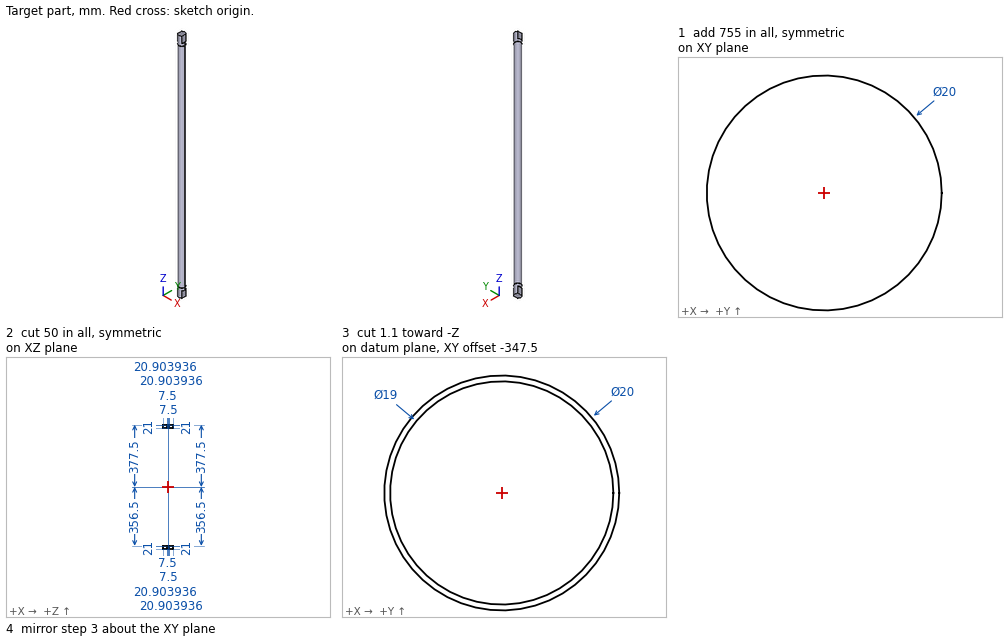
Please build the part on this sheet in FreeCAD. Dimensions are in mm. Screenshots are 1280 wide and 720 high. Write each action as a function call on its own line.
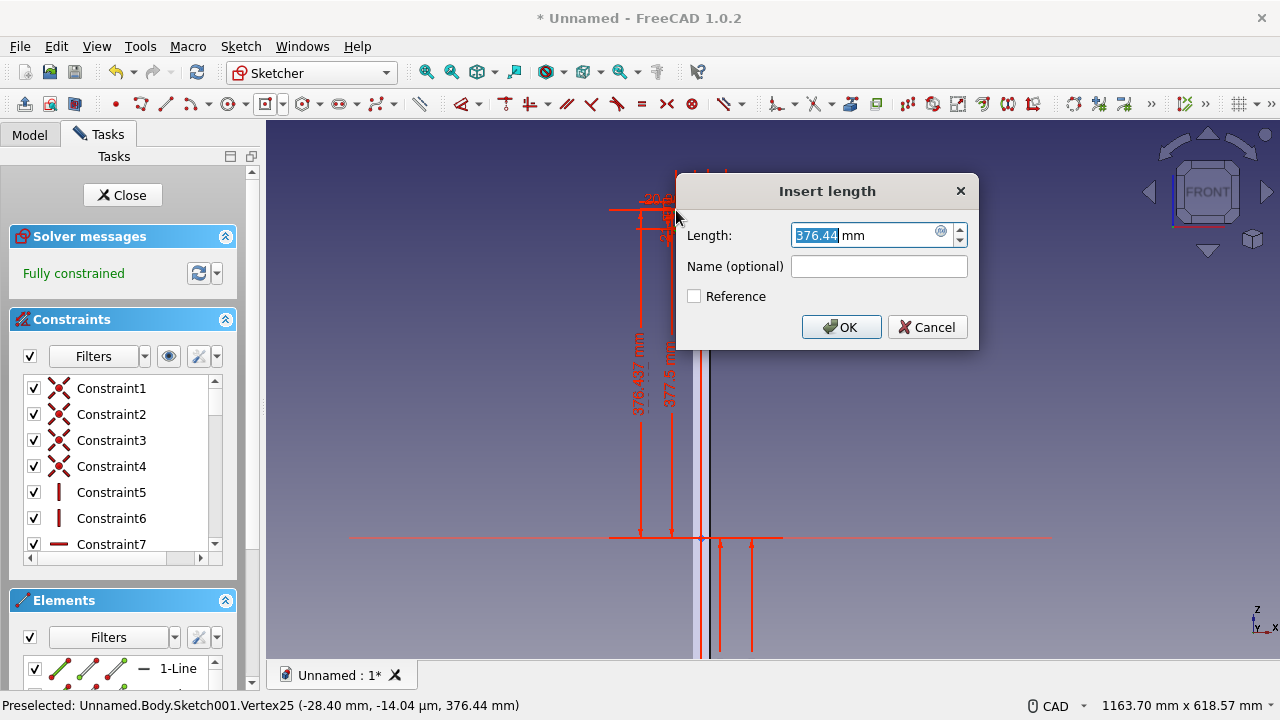
text(377.5)
key(Return)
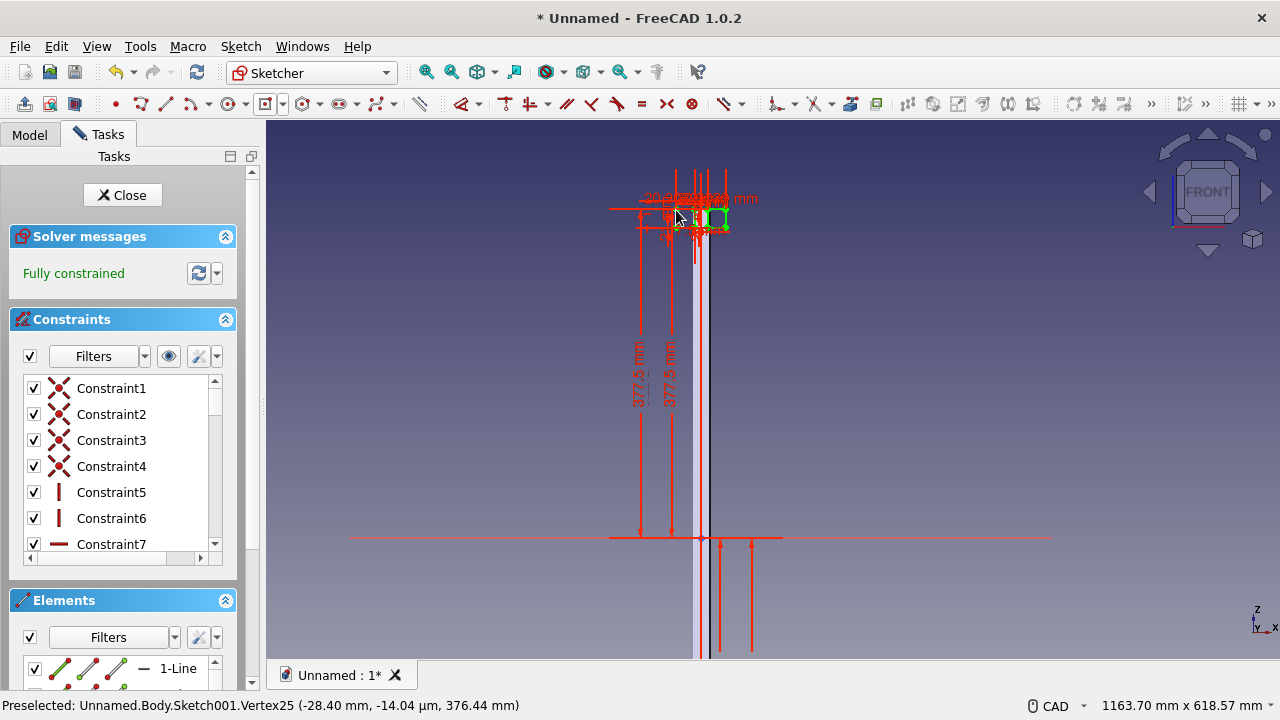
click(123, 195)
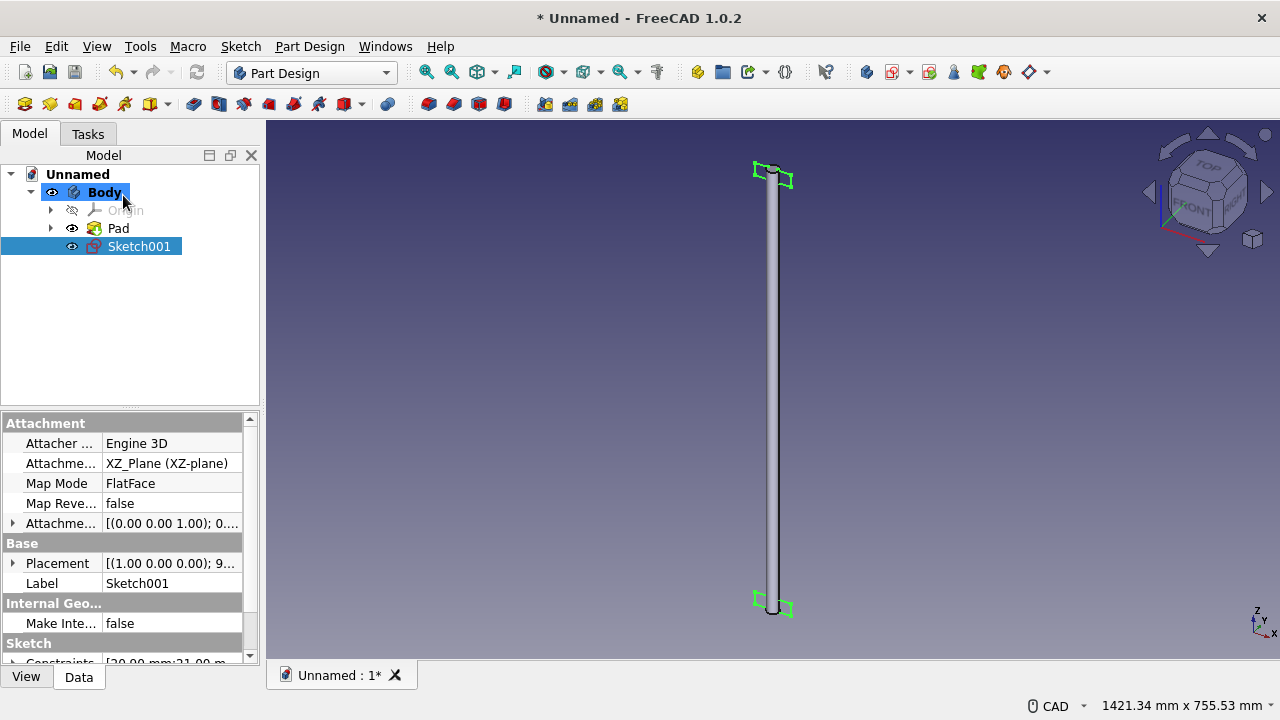
click(194, 104)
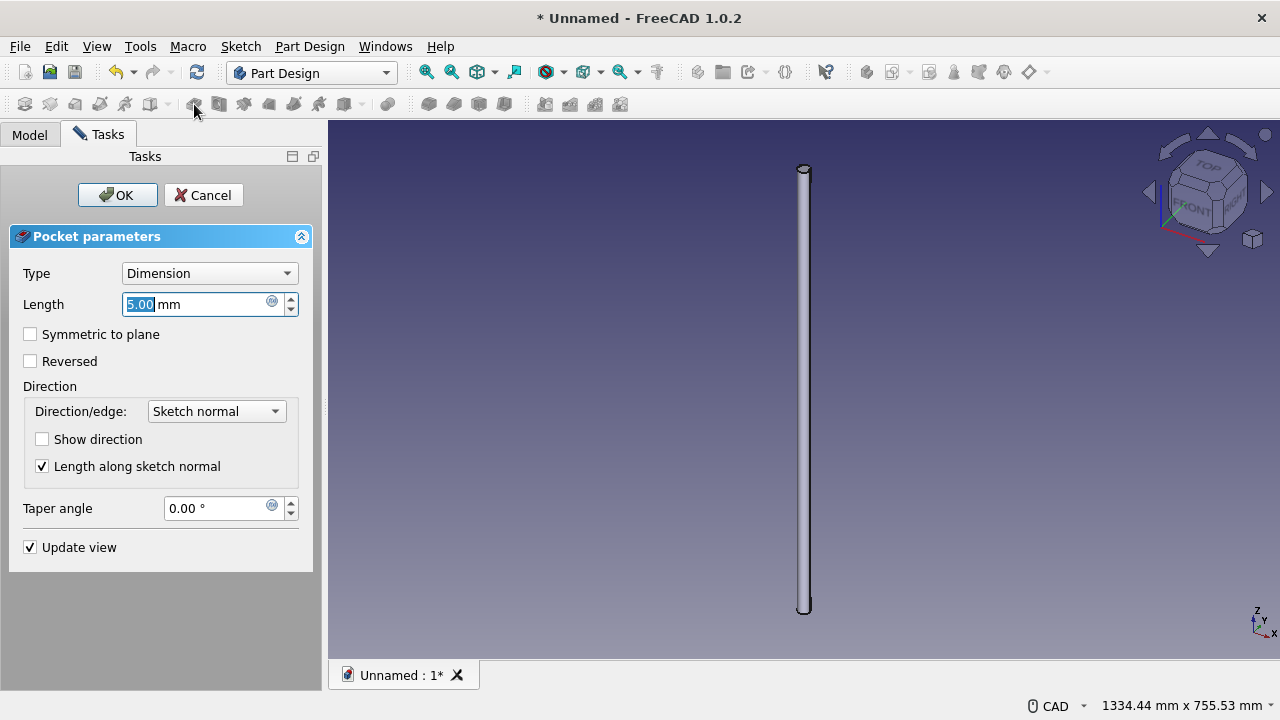
text(50)
key(Tab)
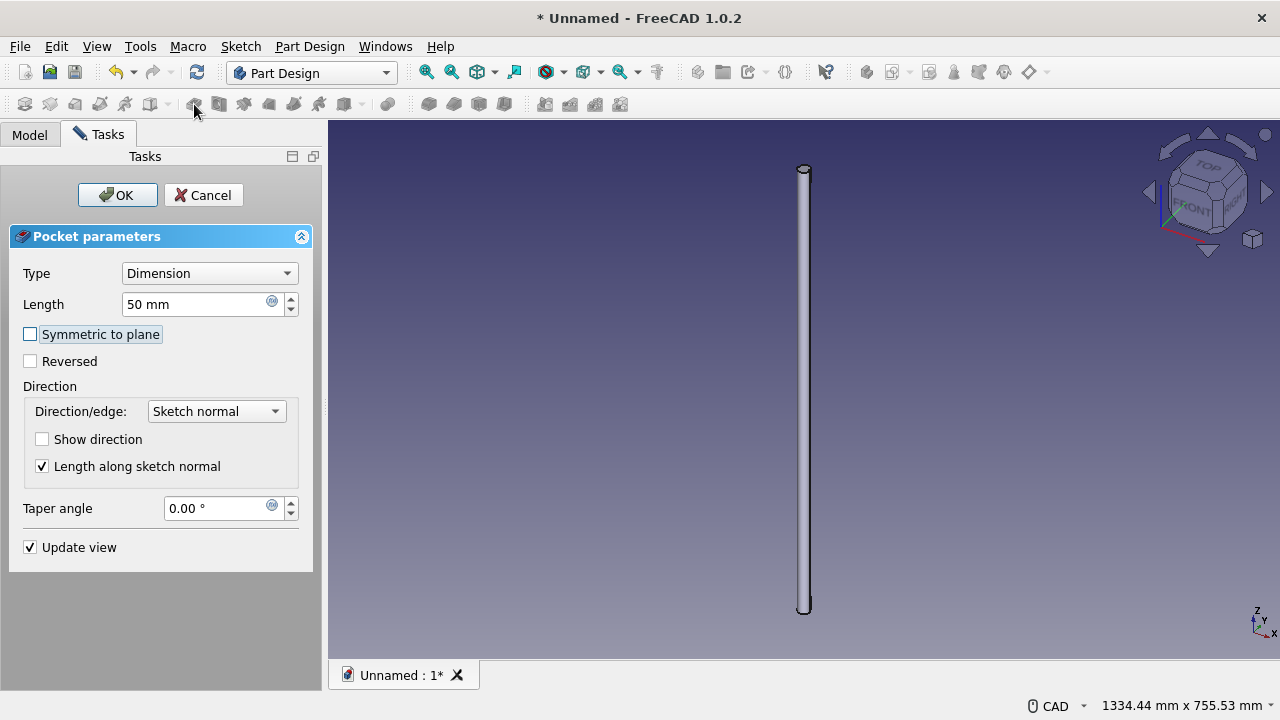
click(31, 334)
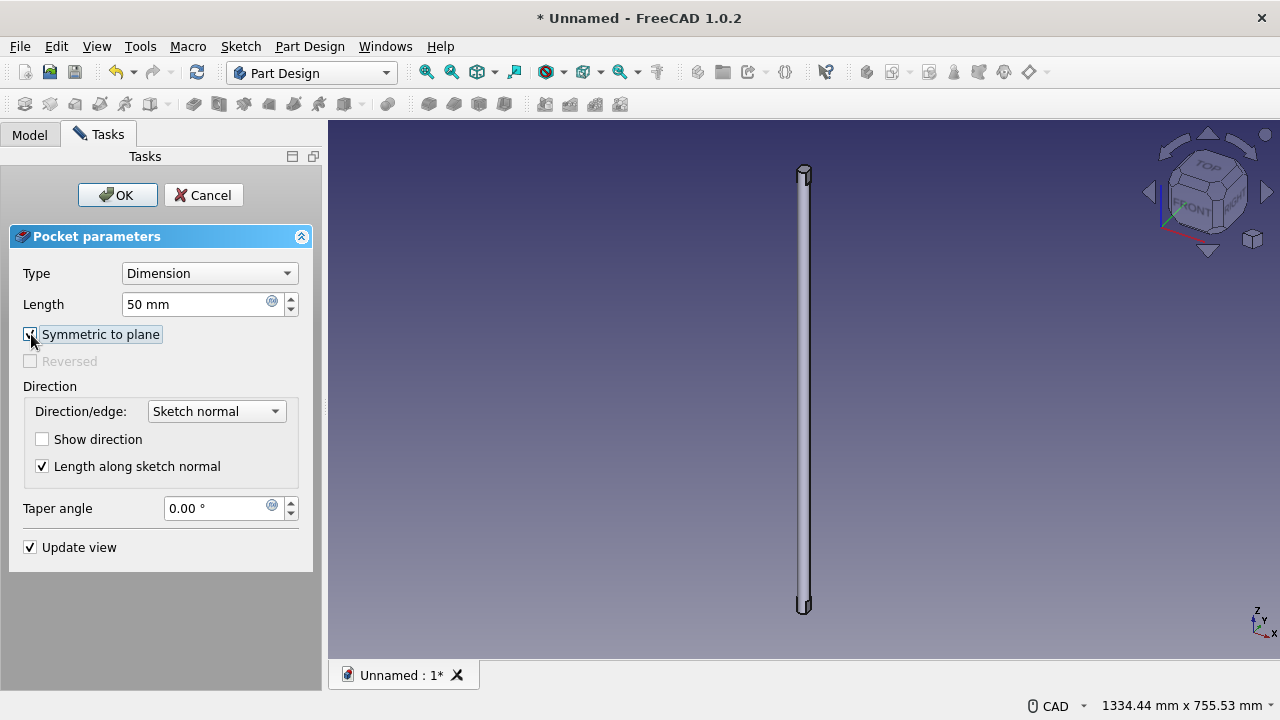
click(118, 195)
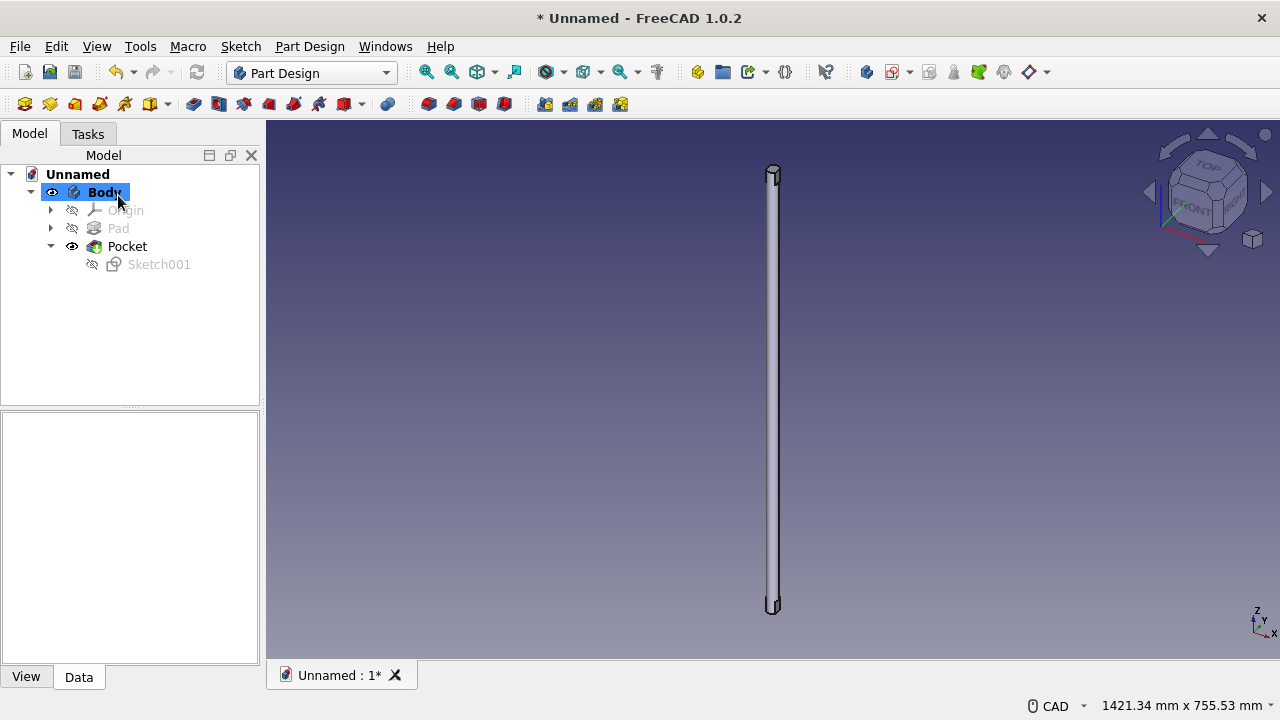
click(51, 210)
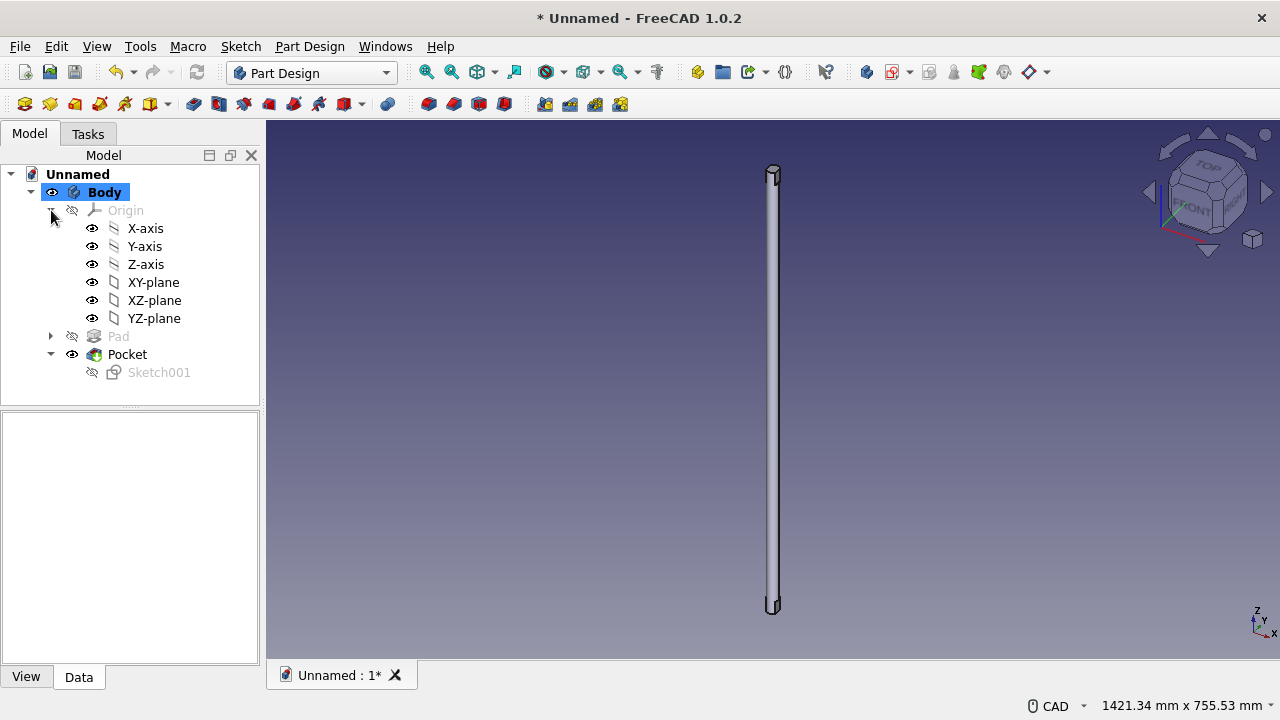
click(137, 282)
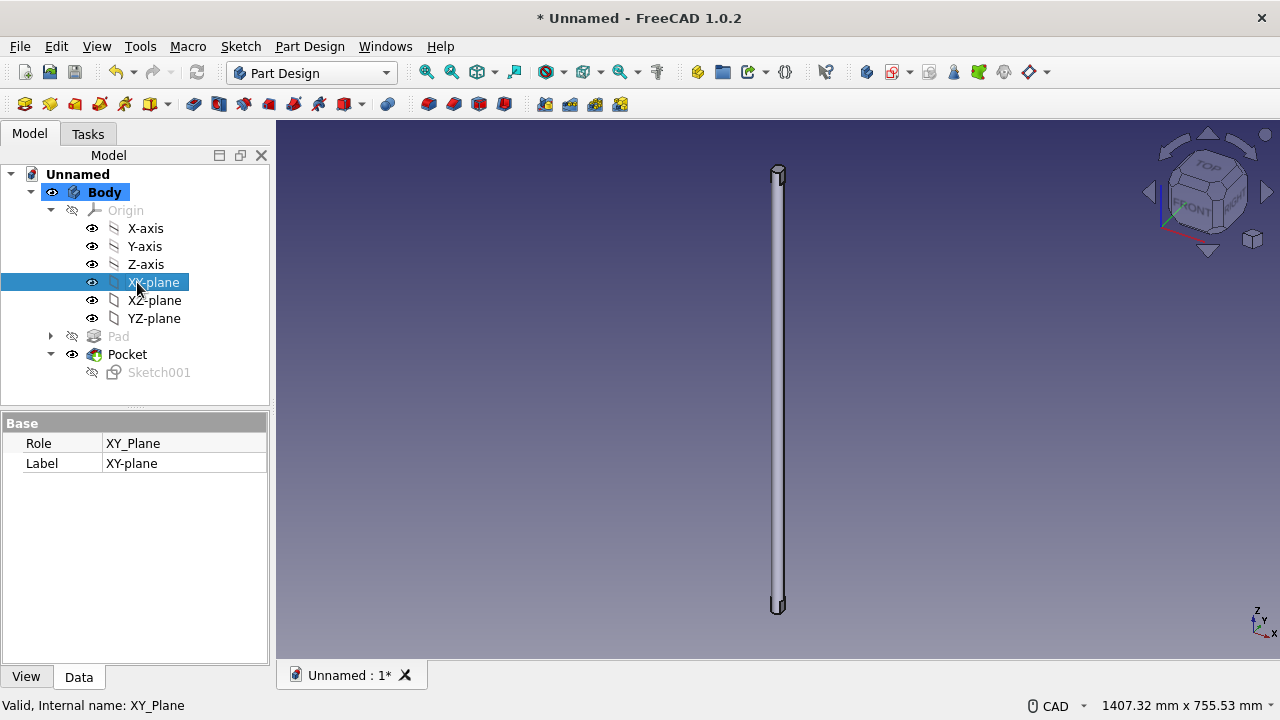
click(1028, 72)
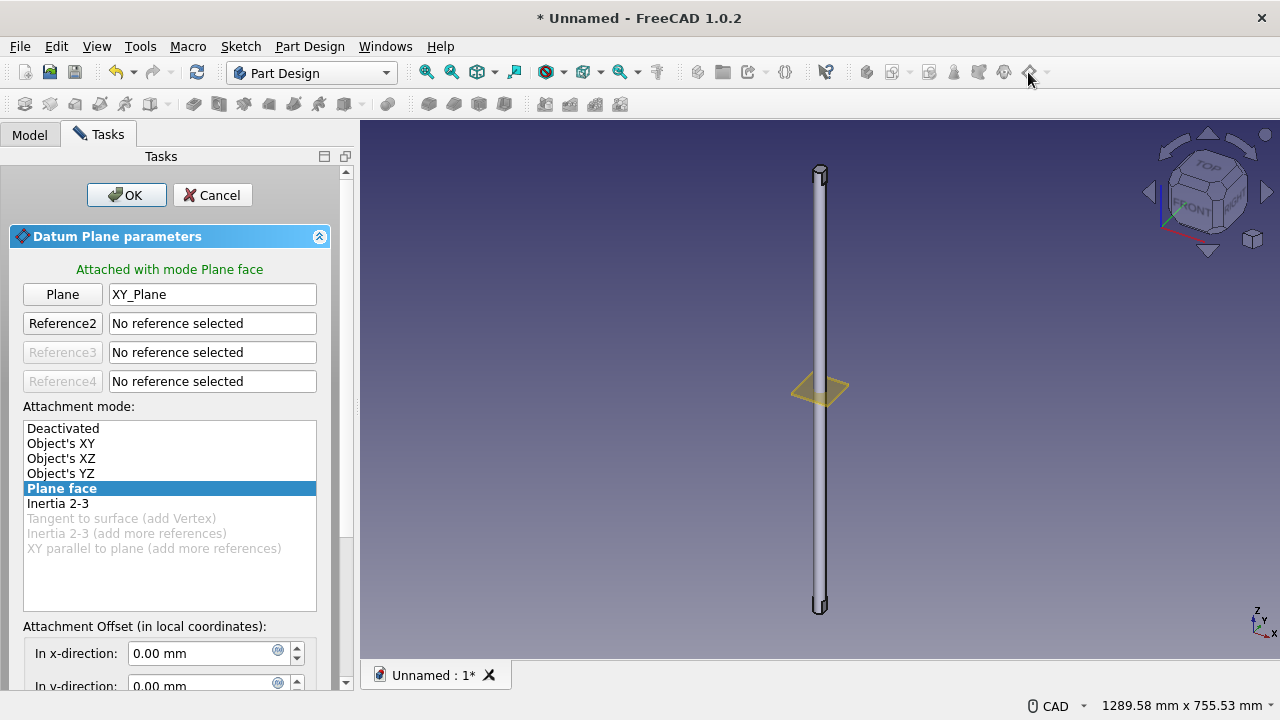
scroll(346, 428, down, 2)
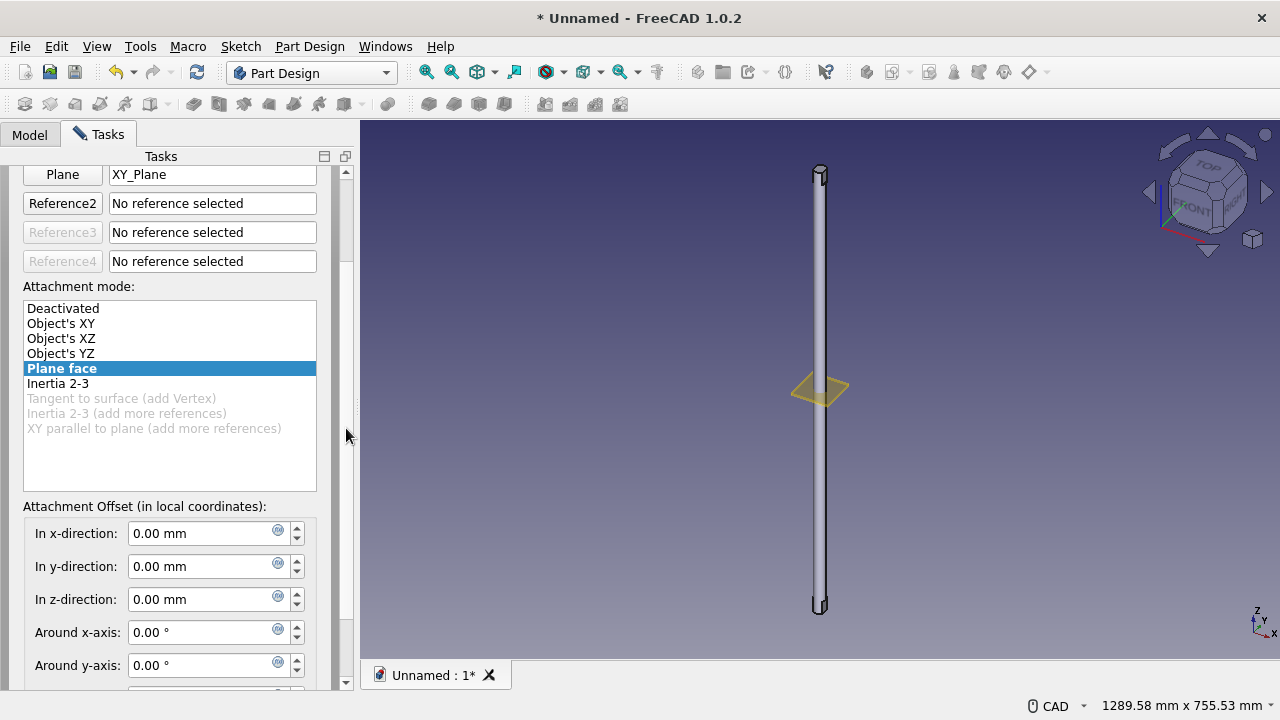
triple_click(210, 600)